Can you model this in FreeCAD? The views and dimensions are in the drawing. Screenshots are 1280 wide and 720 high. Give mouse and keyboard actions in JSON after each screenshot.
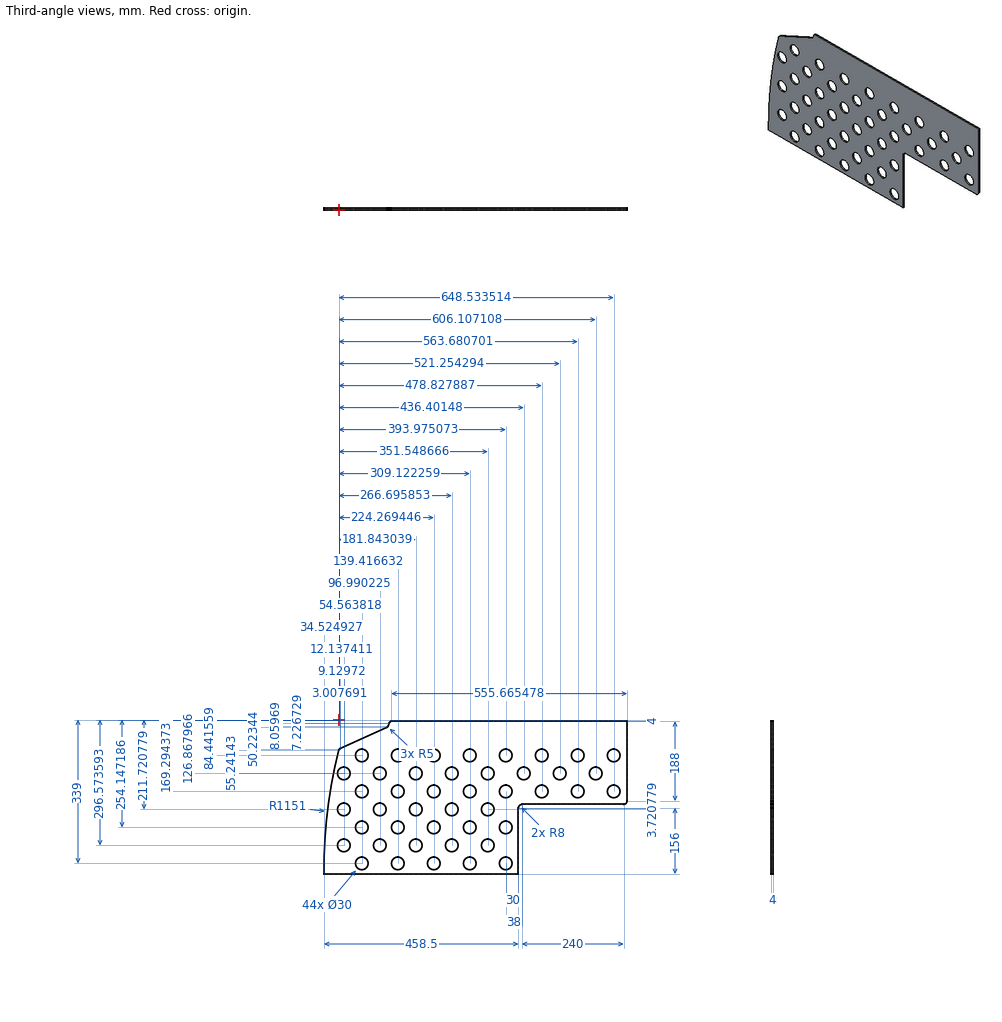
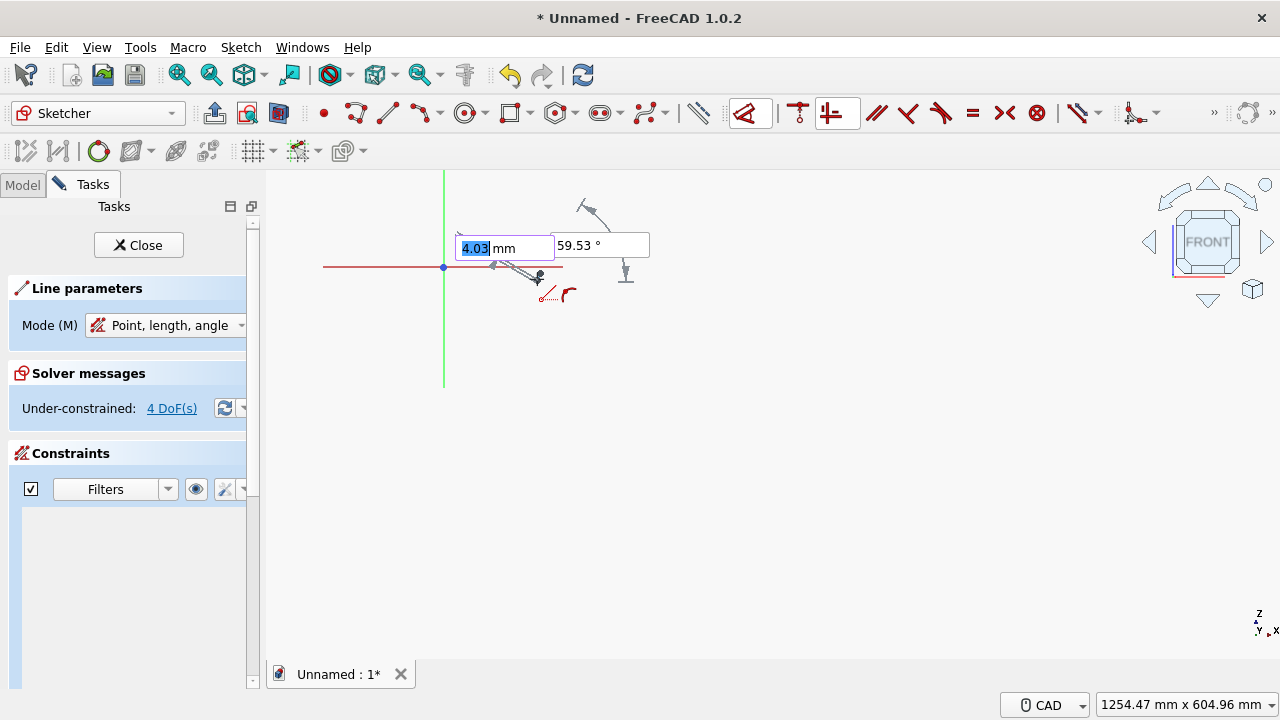
{"action": "scroll", "coordinate": [446, 323], "scroll_direction": "up", "scroll_amount": 10}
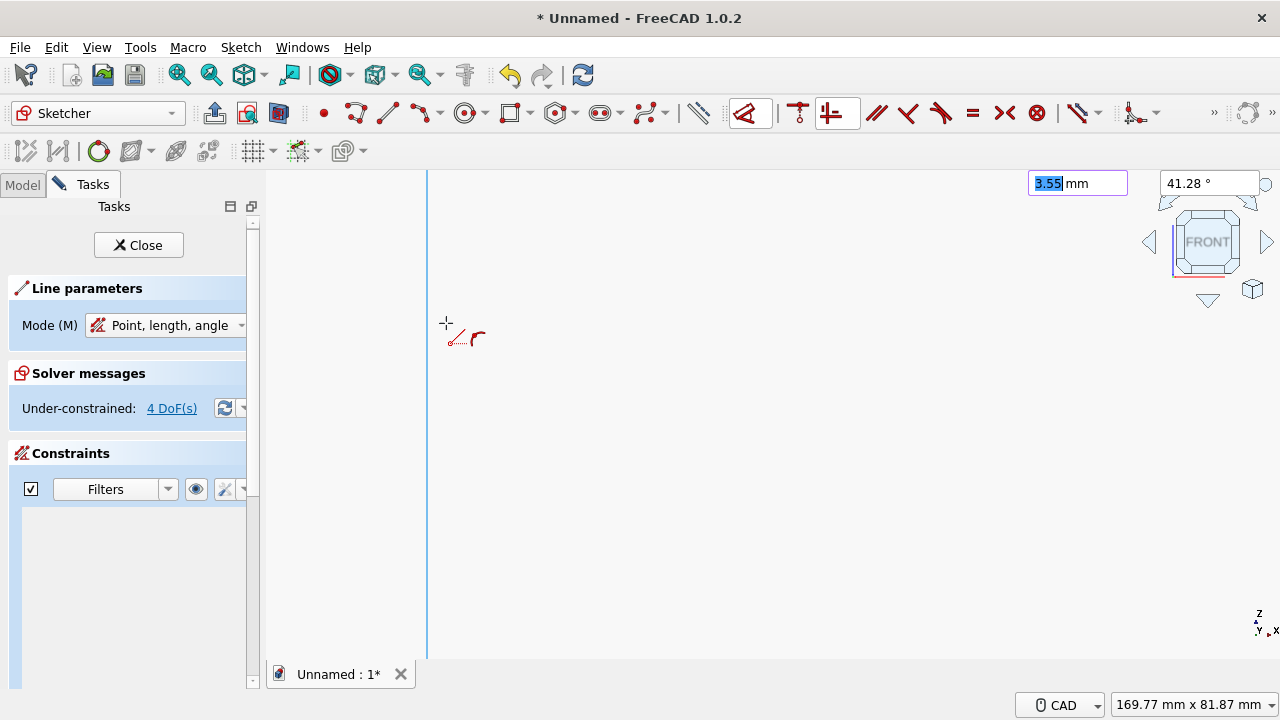
{"action": "left_click", "coordinate": [444, 318]}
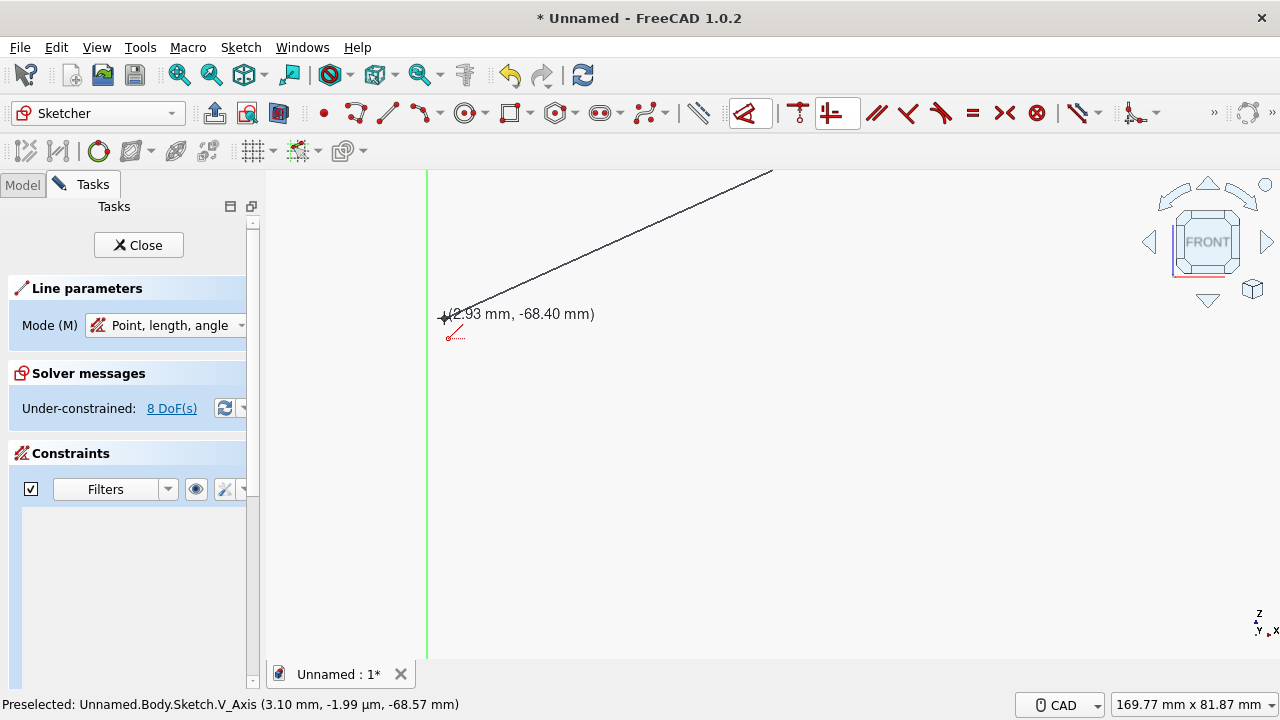
{"action": "left_click", "coordinate": [356, 114]}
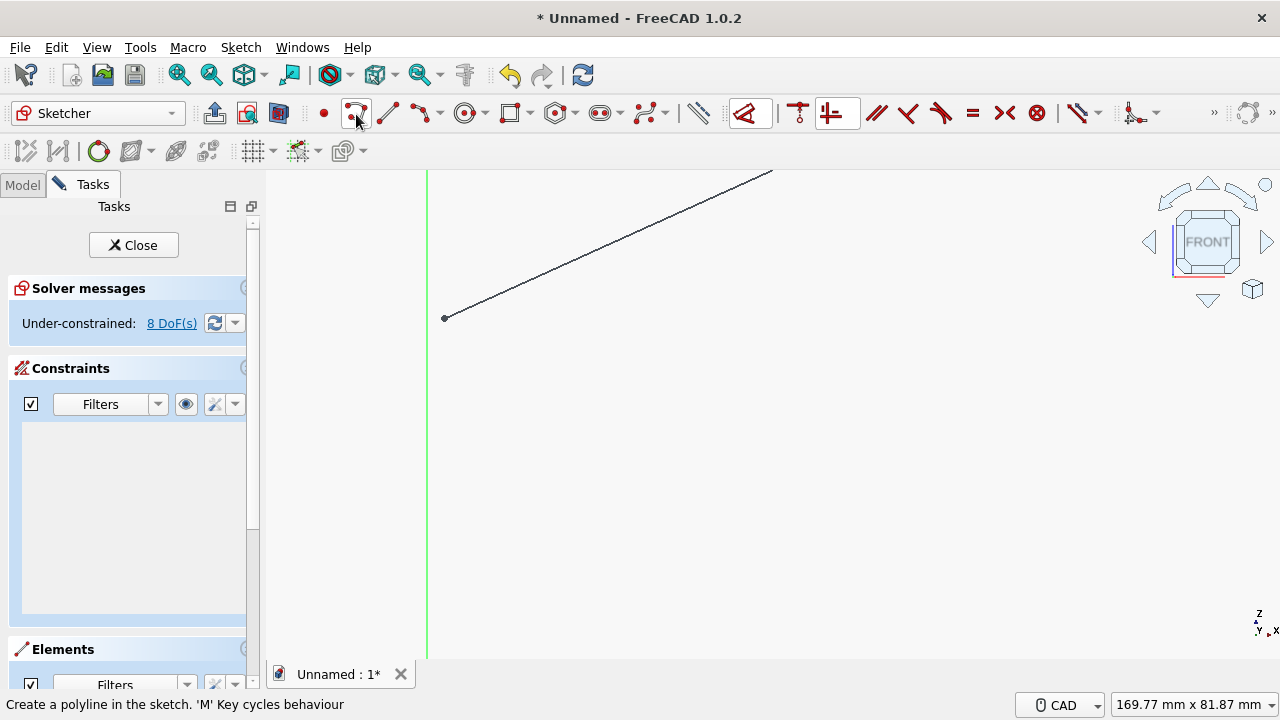
{"action": "scroll", "coordinate": [446, 323], "scroll_direction": "down", "scroll_amount": 10}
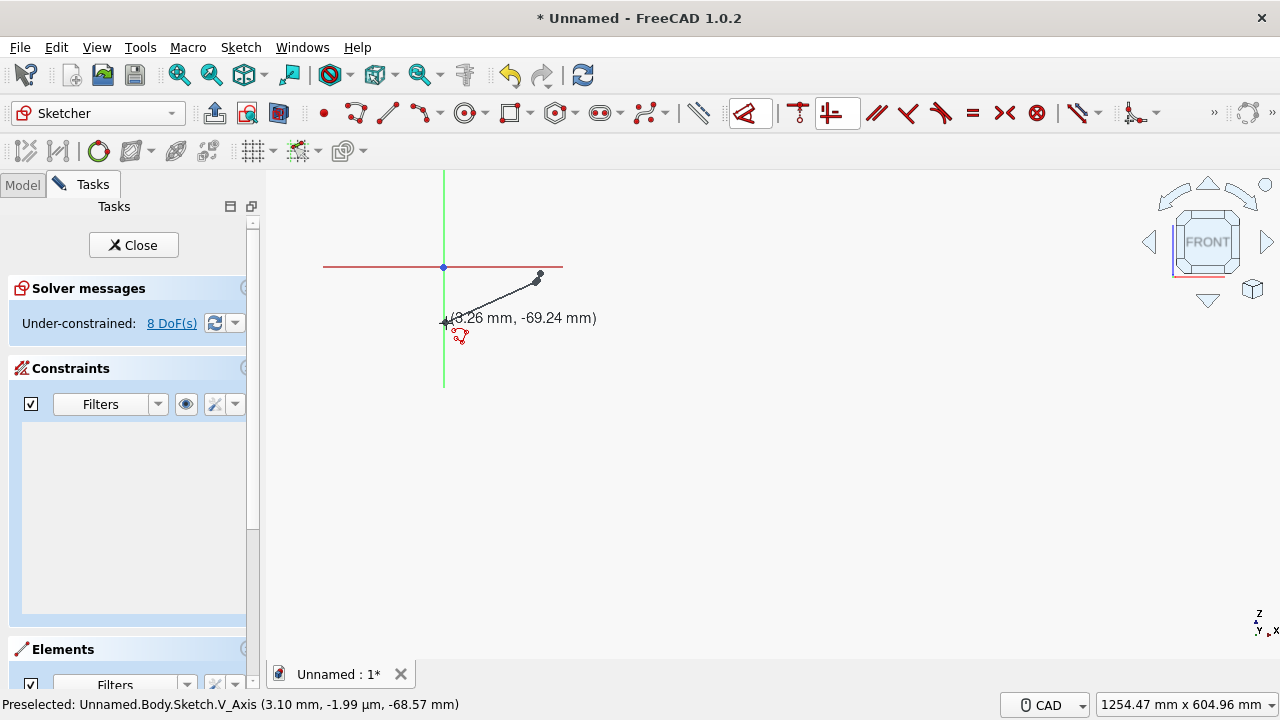
{"action": "left_click", "coordinate": [416, 562]}
{"action": "left_click", "coordinate": [786, 562]}
{"action": "left_click", "coordinate": [786, 436]}
{"action": "right_click", "coordinate": [786, 436]}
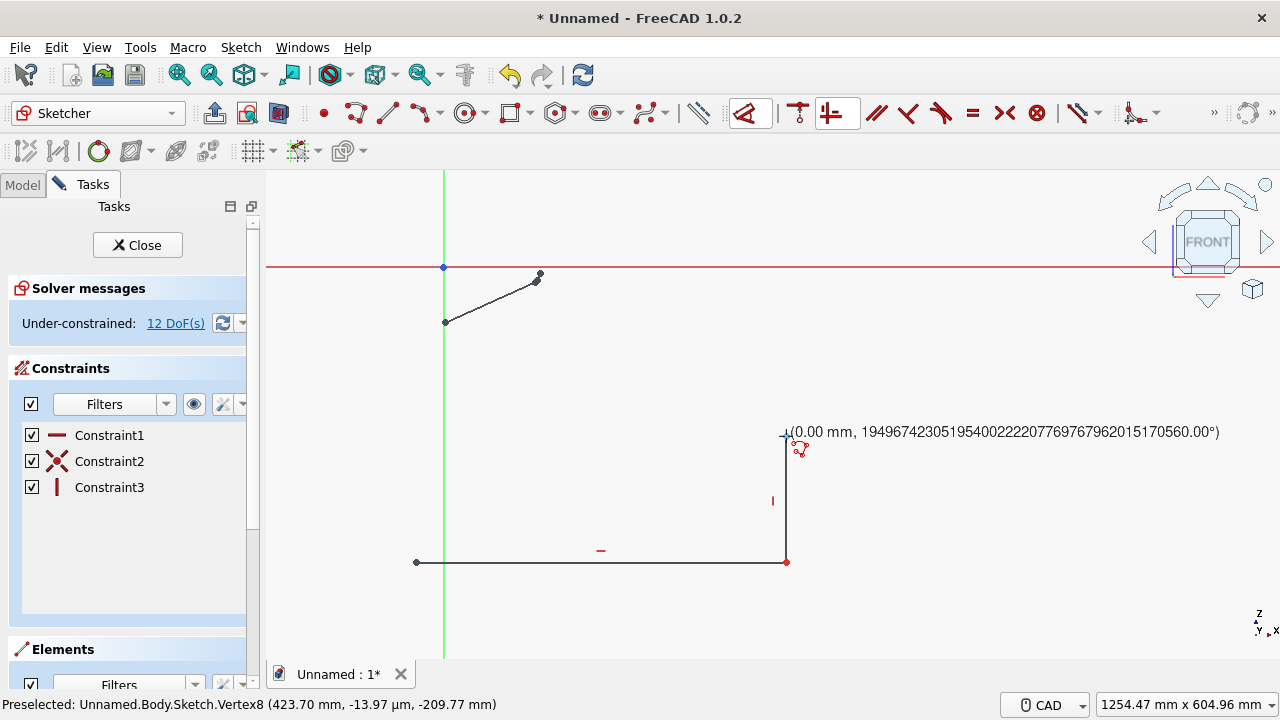
{"action": "key", "text": "g l"}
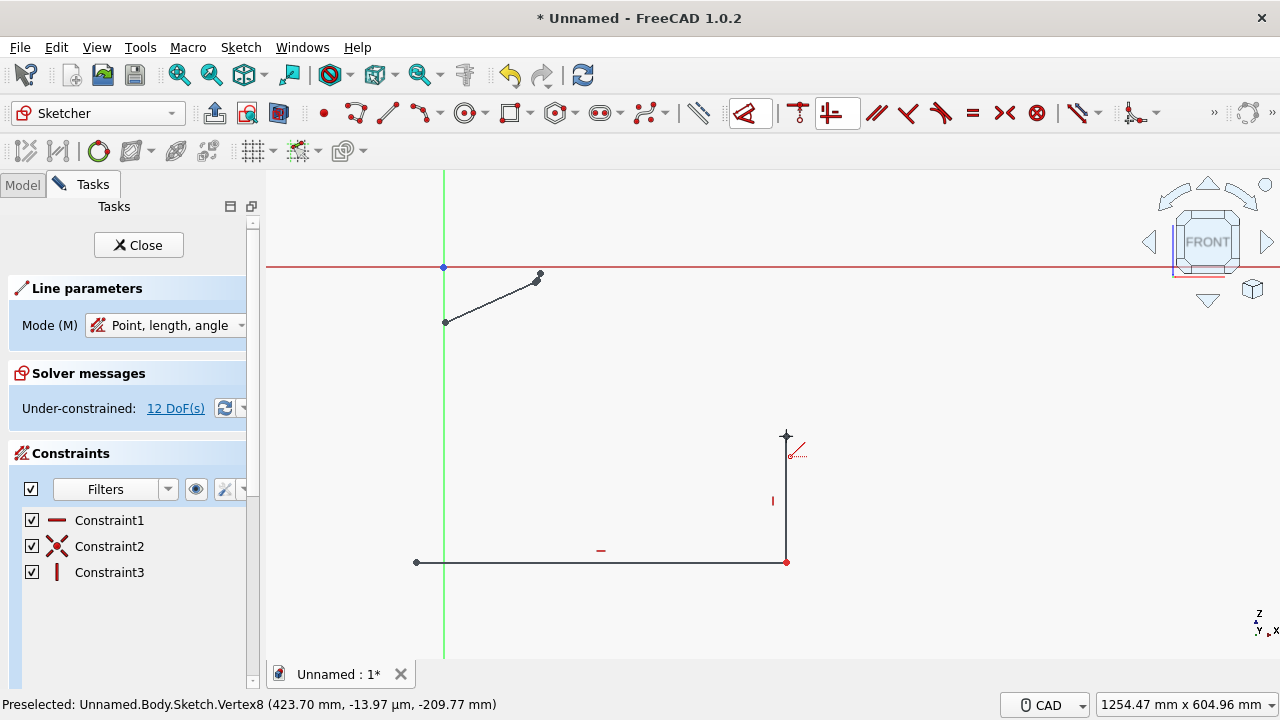
{"action": "scroll", "coordinate": [793, 429], "scroll_direction": "up", "scroll_amount": 3}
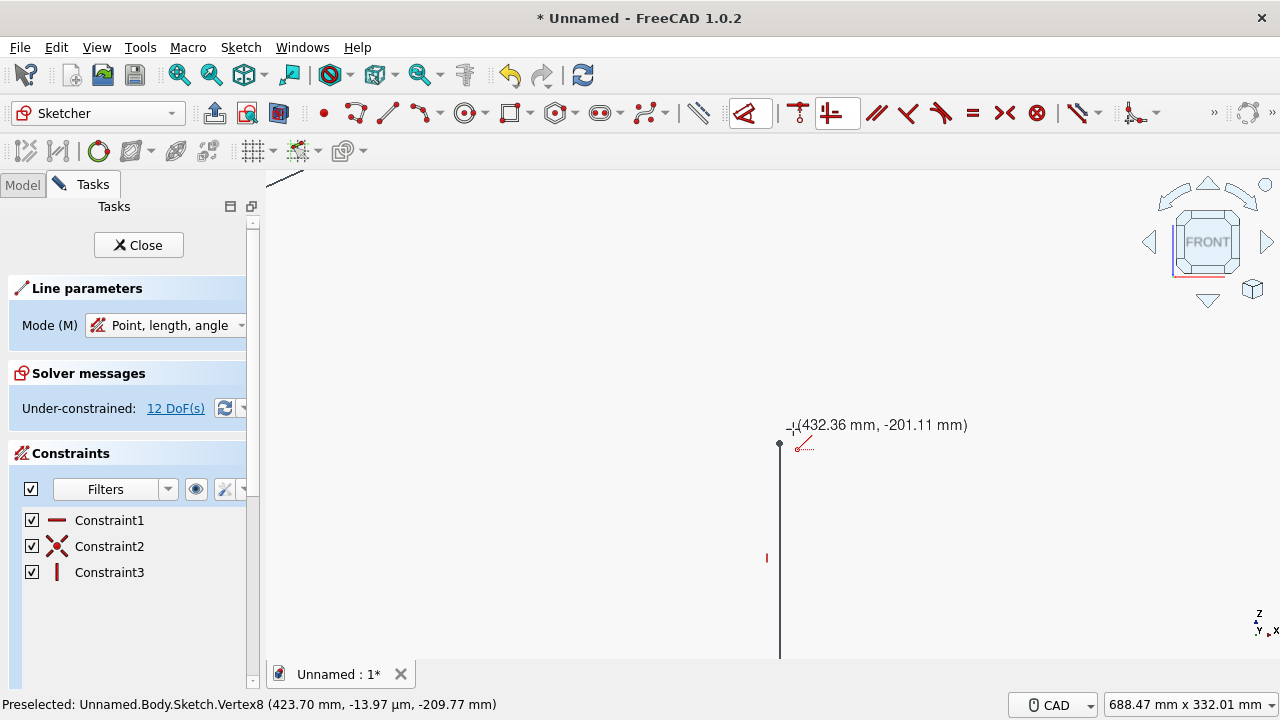
{"action": "left_click", "coordinate": [792, 429]}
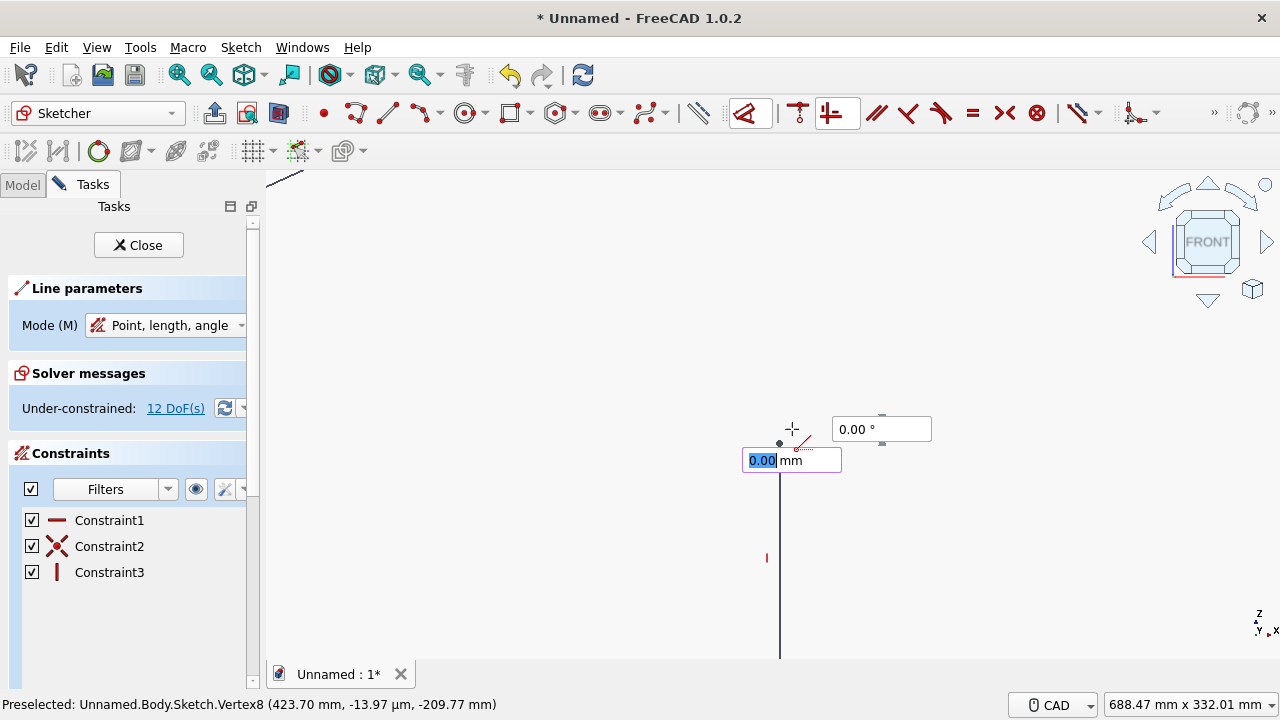
{"action": "scroll", "coordinate": [794, 429], "scroll_direction": "down", "scroll_amount": 3}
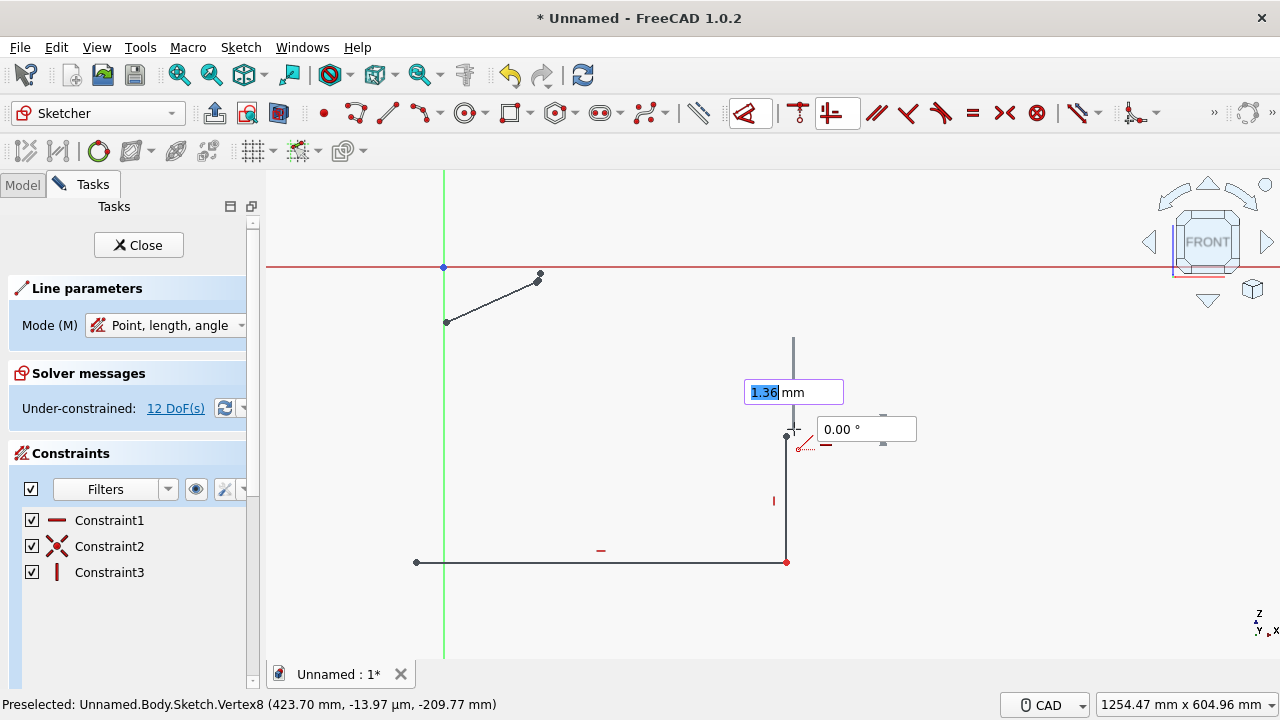
{"action": "left_click", "coordinate": [987, 429]}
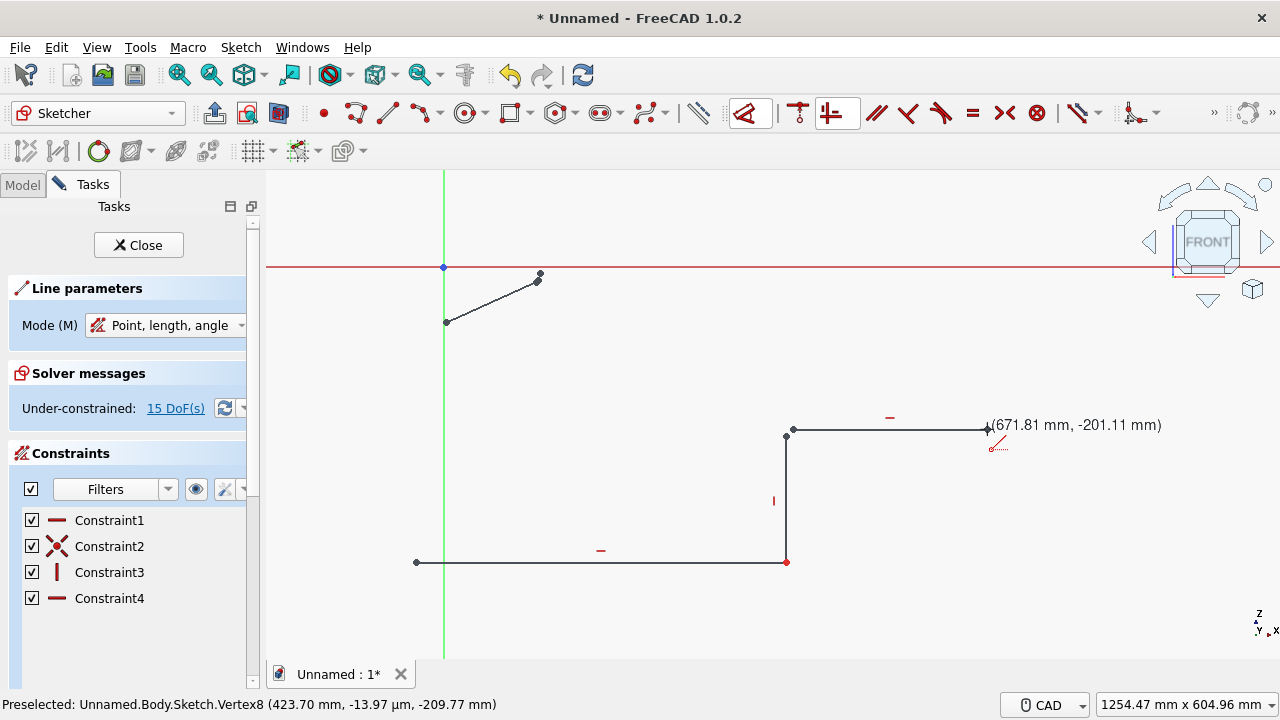
{"action": "key", "text": "g m"}